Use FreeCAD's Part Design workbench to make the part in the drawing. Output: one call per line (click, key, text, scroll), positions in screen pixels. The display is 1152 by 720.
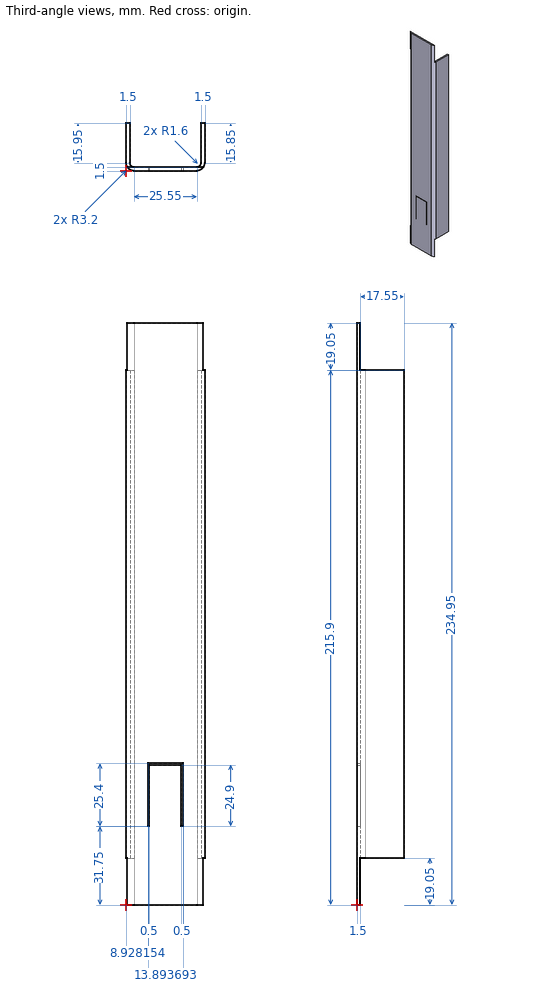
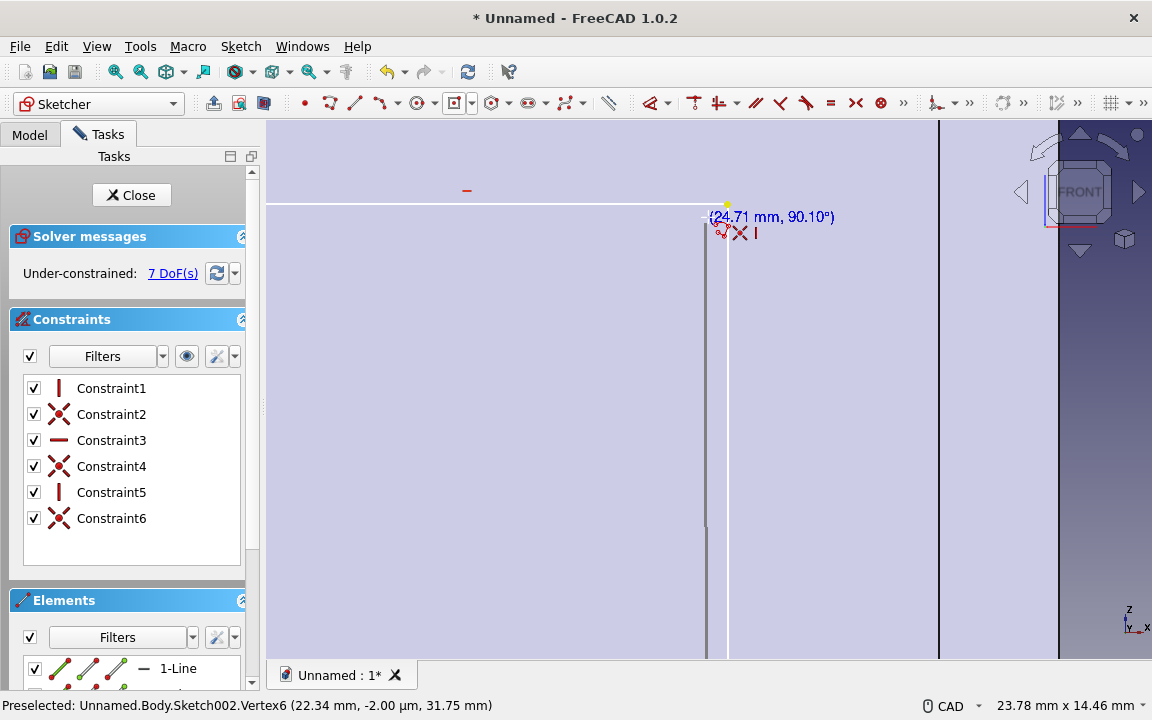
click(707, 216)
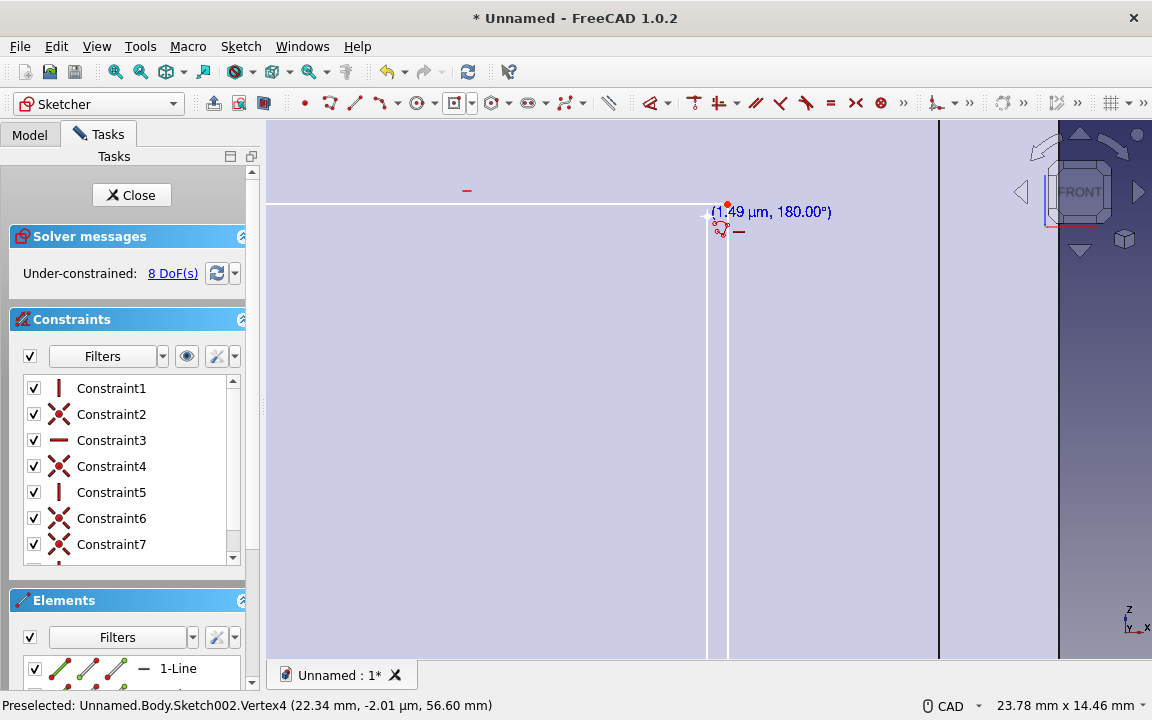
scroll(708, 217, down, 9)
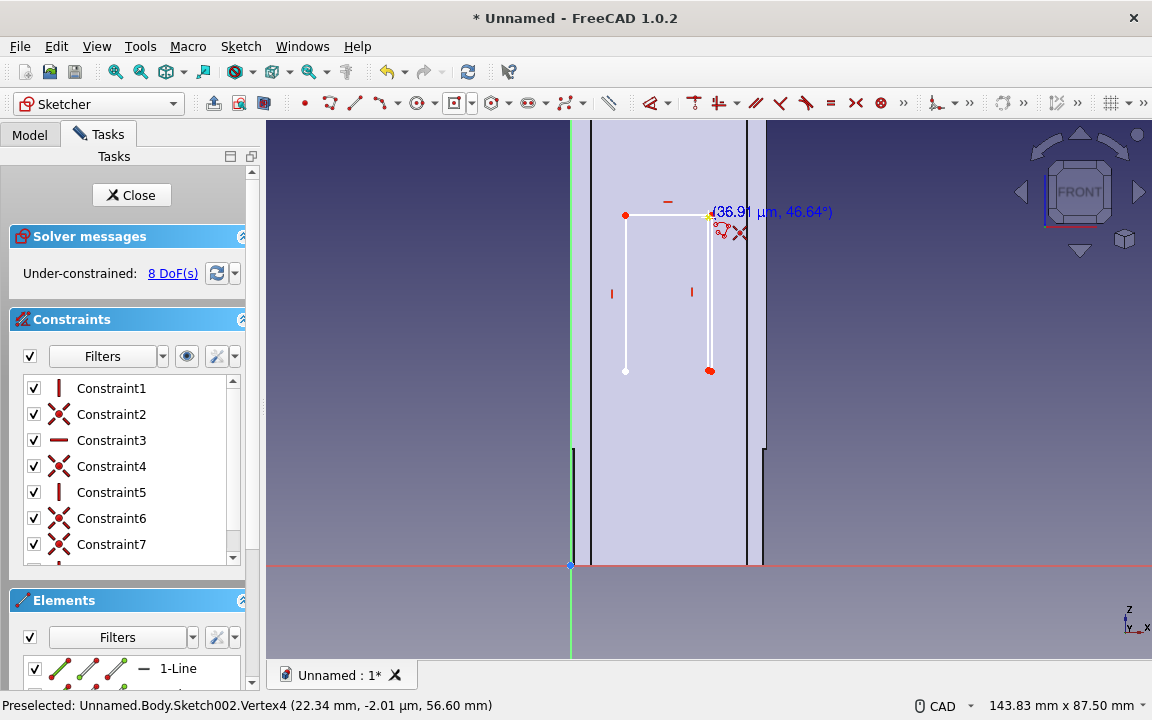
scroll(629, 217, up, 9)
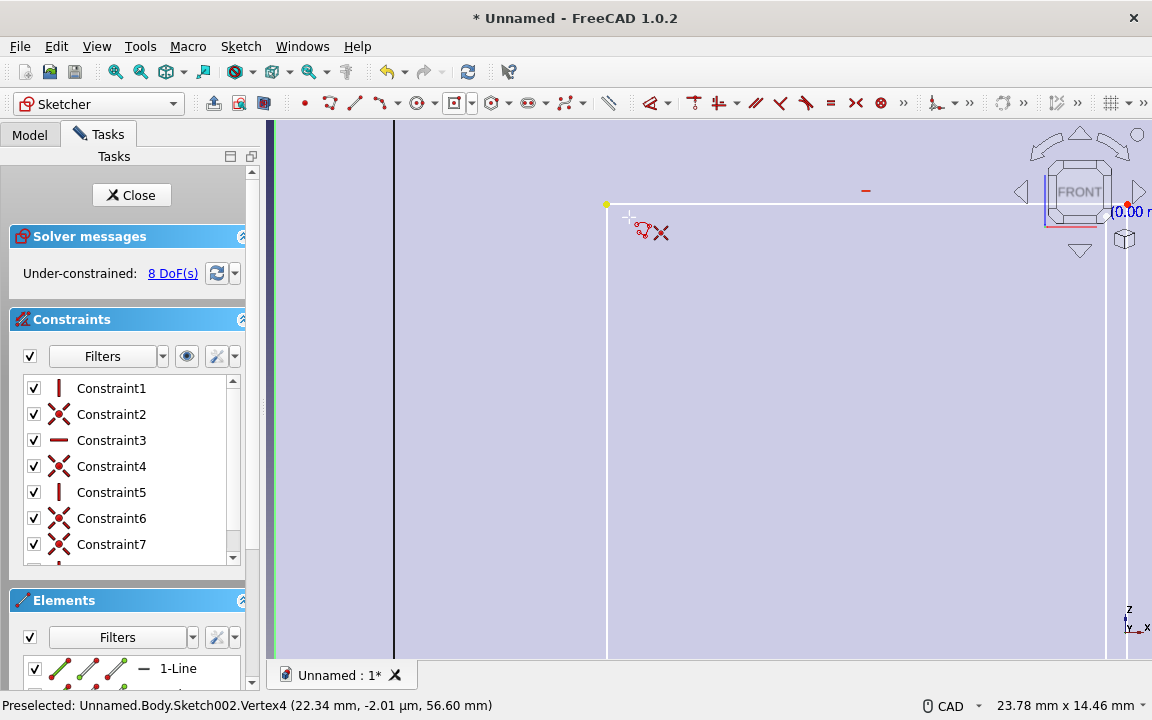
click(626, 216)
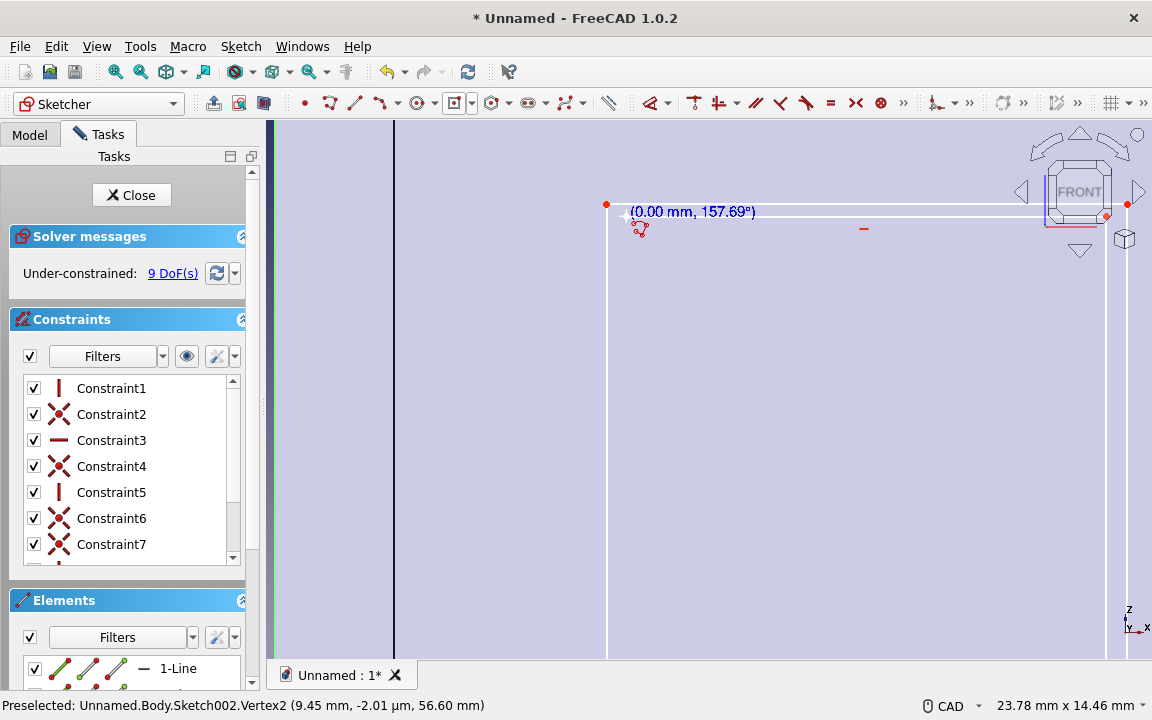
scroll(629, 217, down, 9)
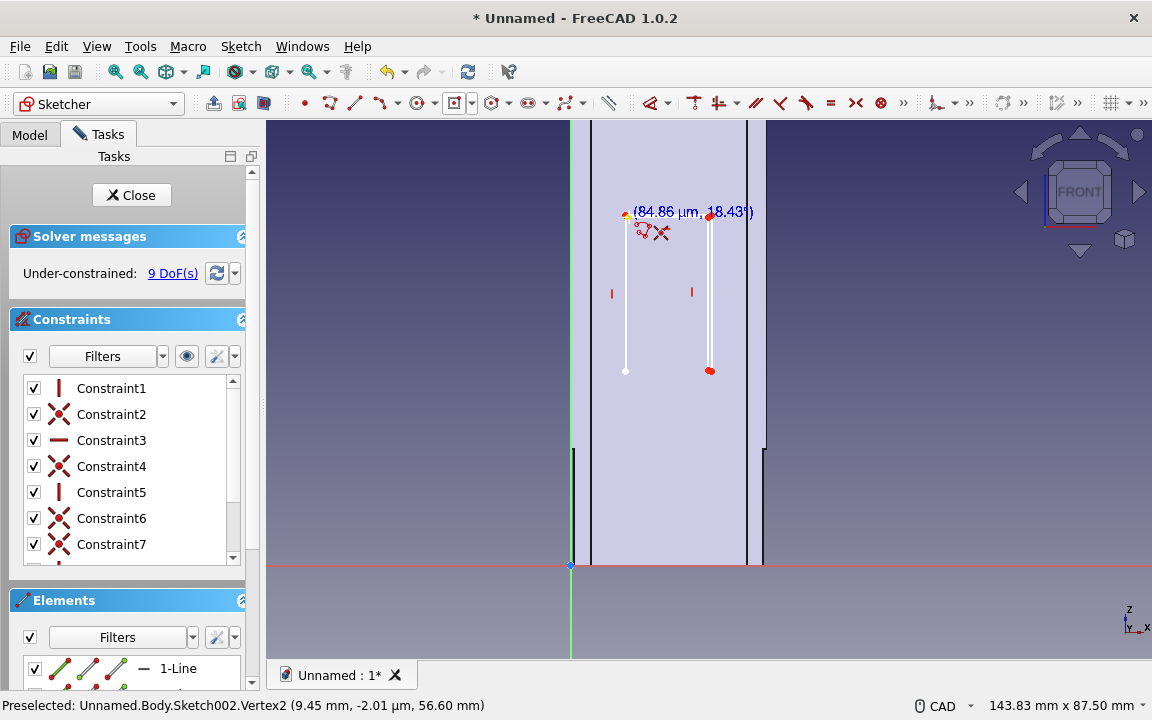
scroll(629, 370, up, 9)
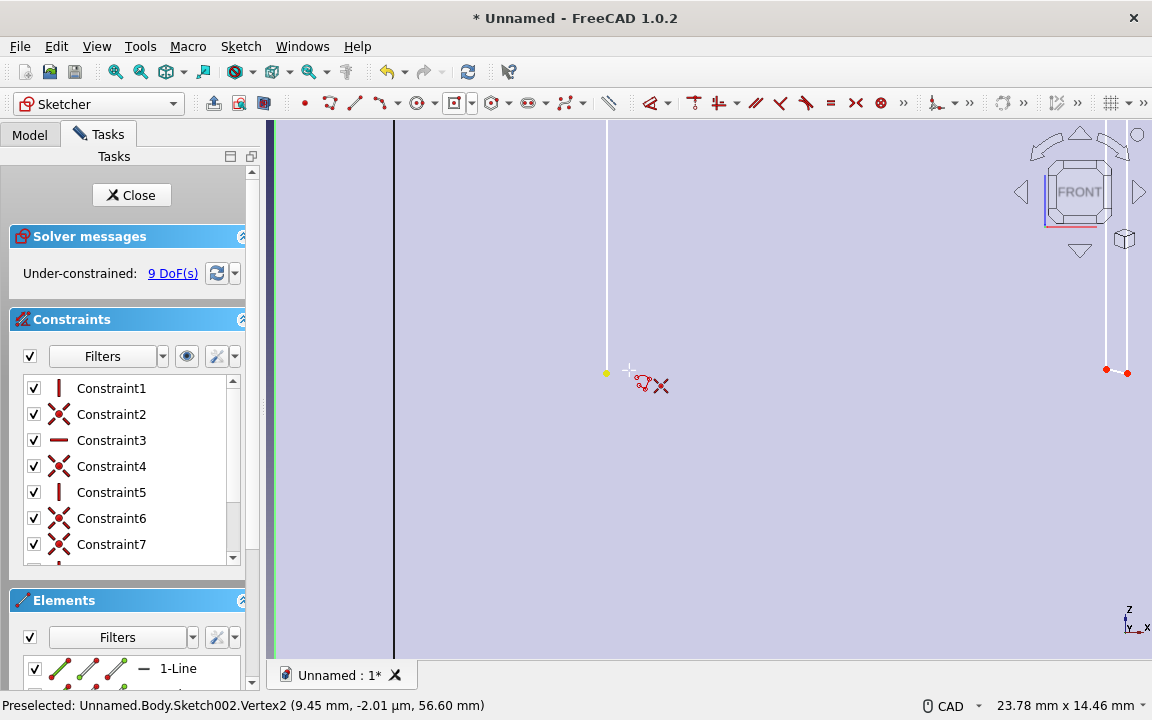
click(626, 370)
click(607, 374)
key(Escape)
key(Escape)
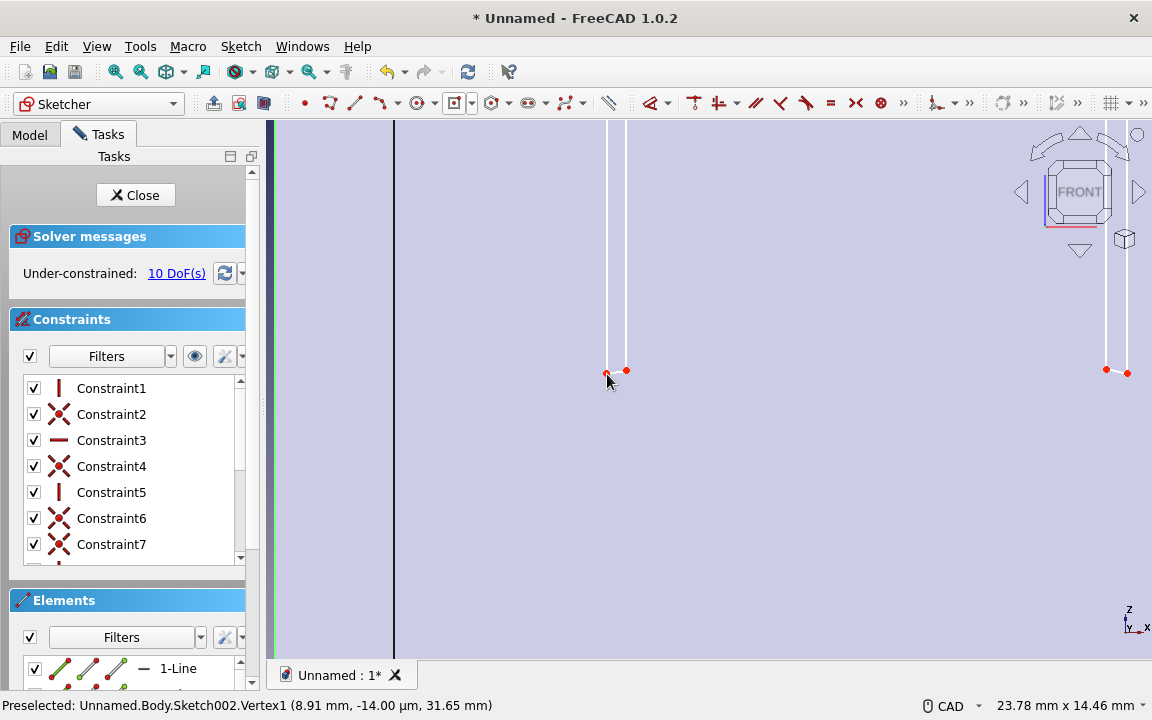
scroll(629, 370, down, 9)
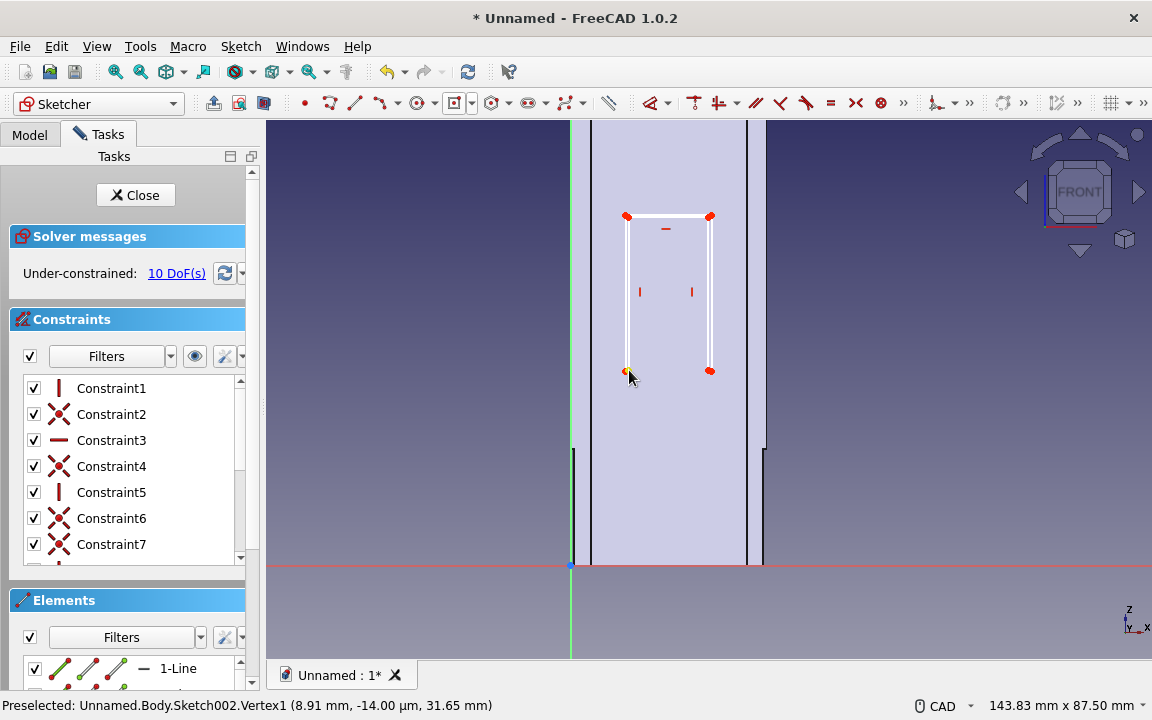
scroll(710, 371, up, 11)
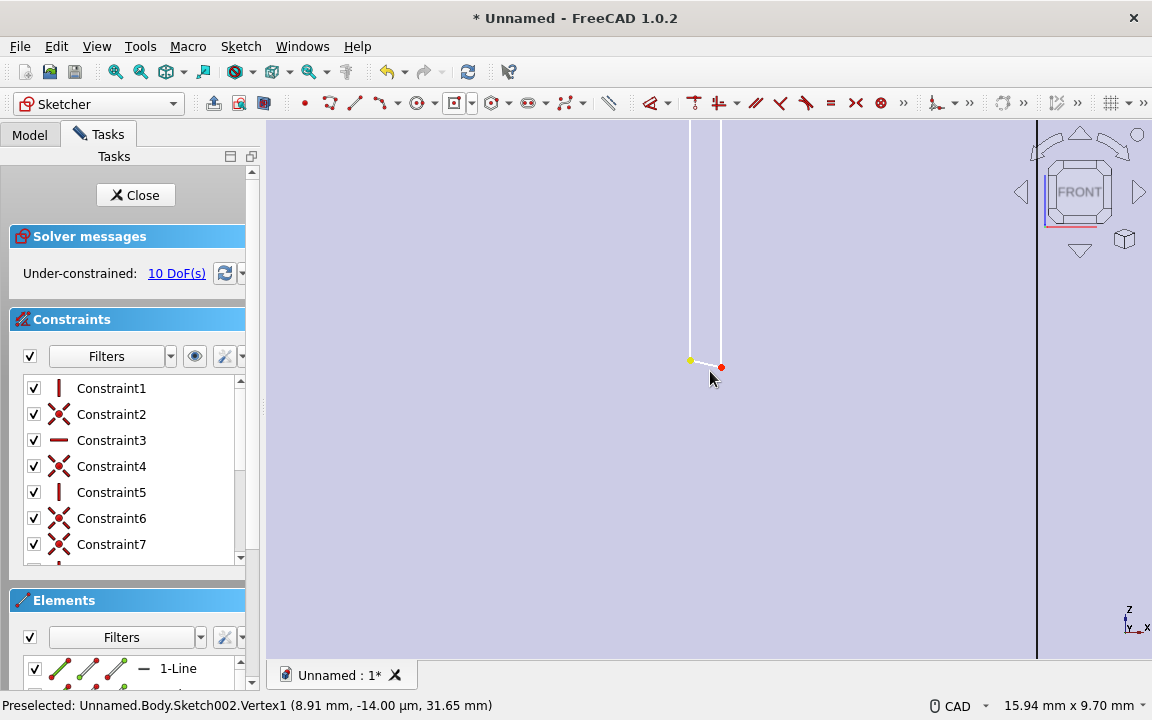
click(706, 364)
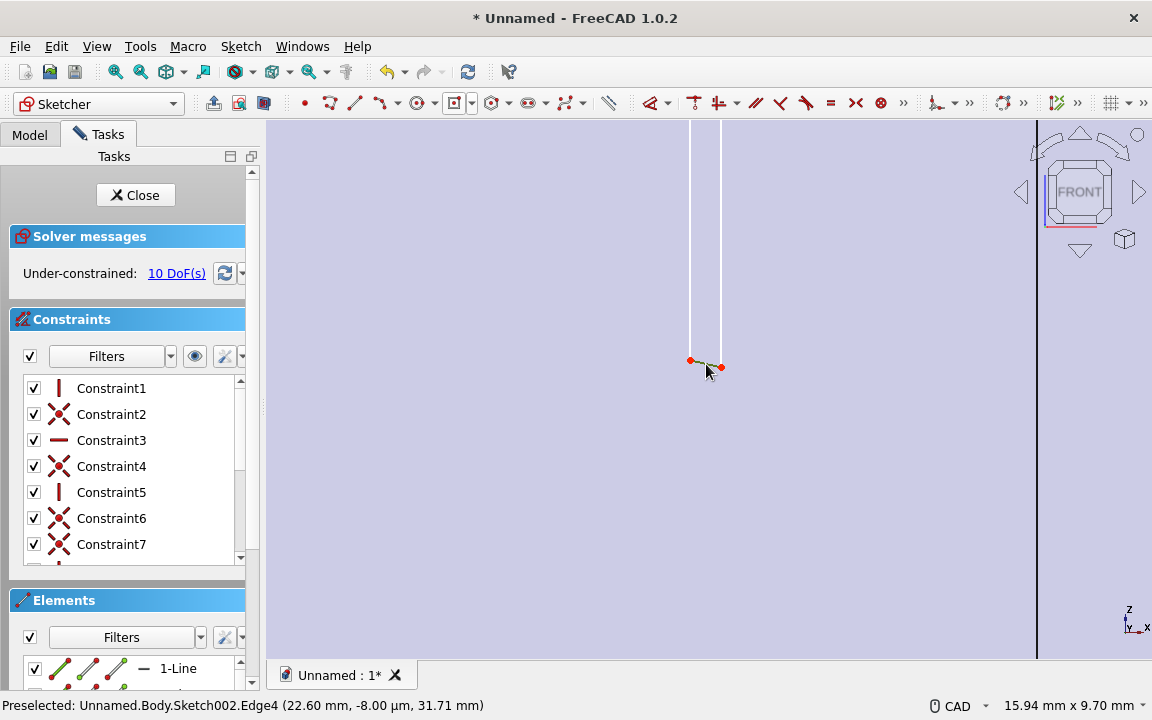
key(h)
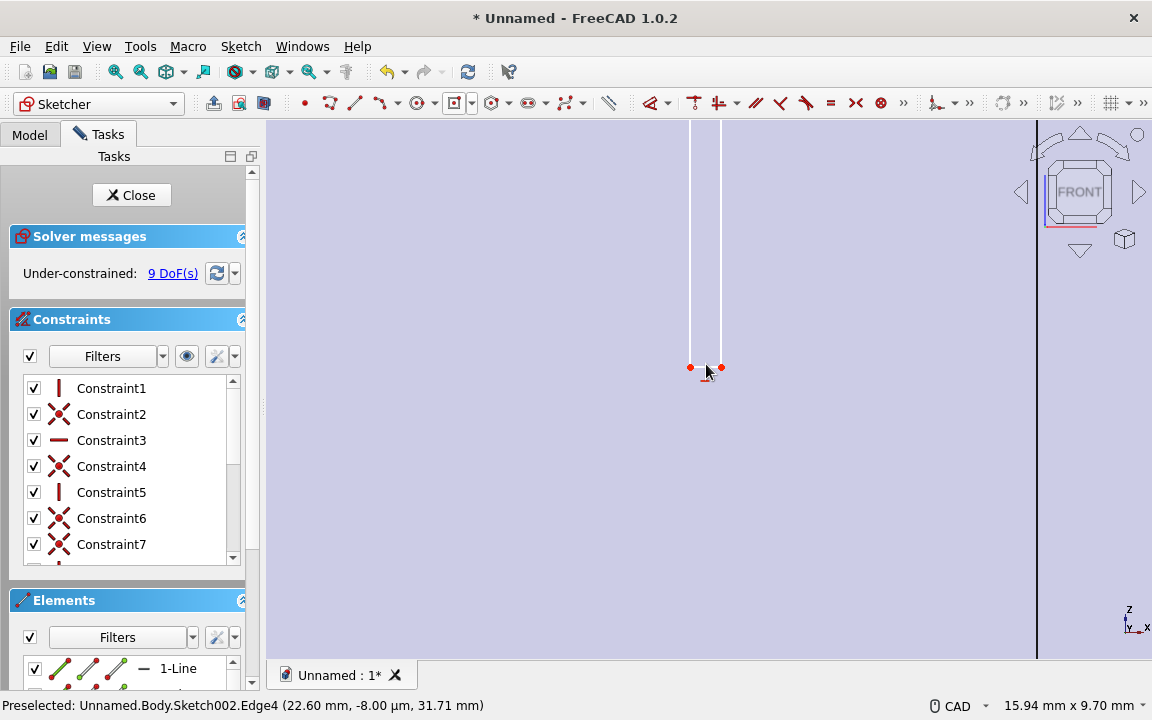
scroll(710, 371, down, 11)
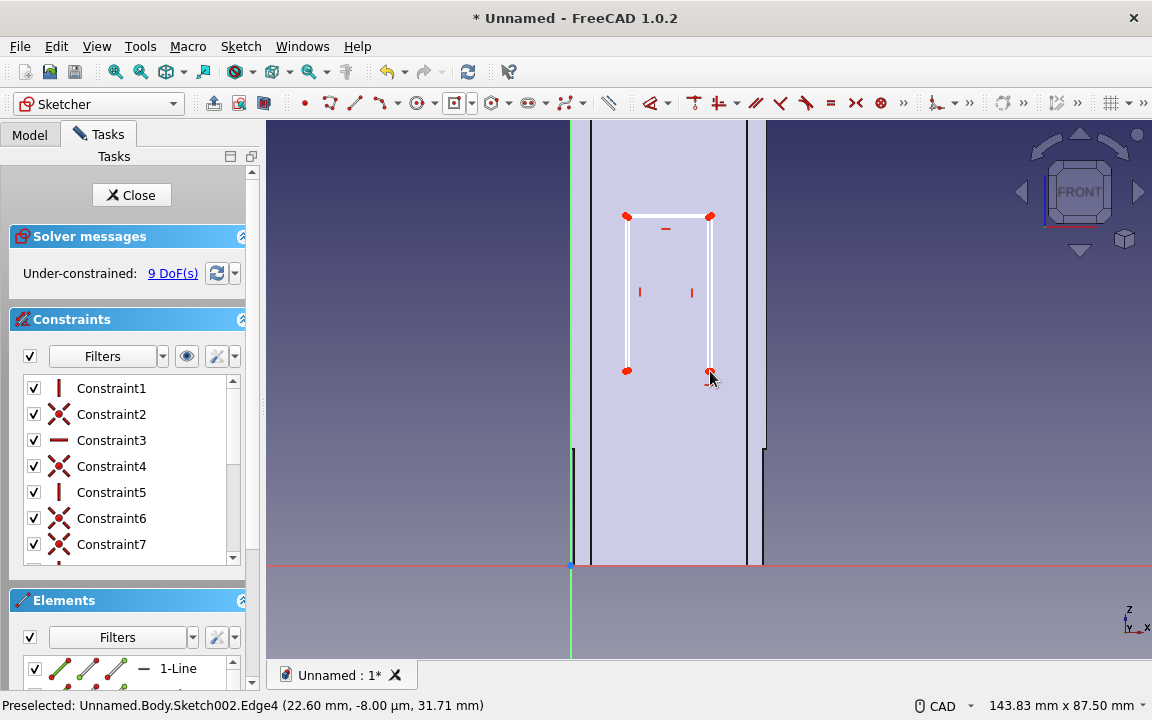
scroll(628, 371, up, 12)